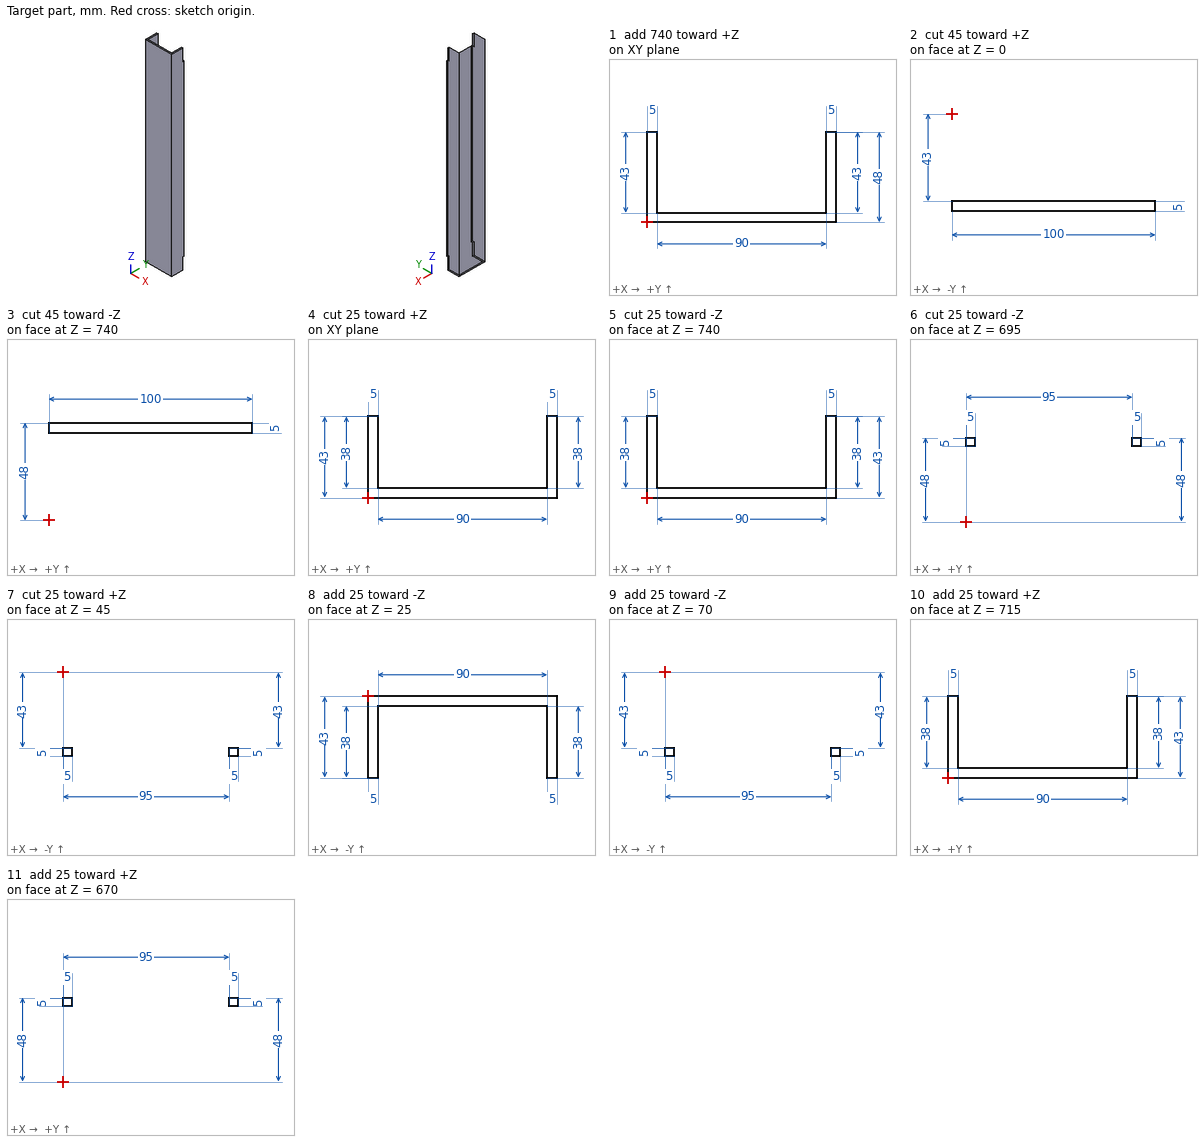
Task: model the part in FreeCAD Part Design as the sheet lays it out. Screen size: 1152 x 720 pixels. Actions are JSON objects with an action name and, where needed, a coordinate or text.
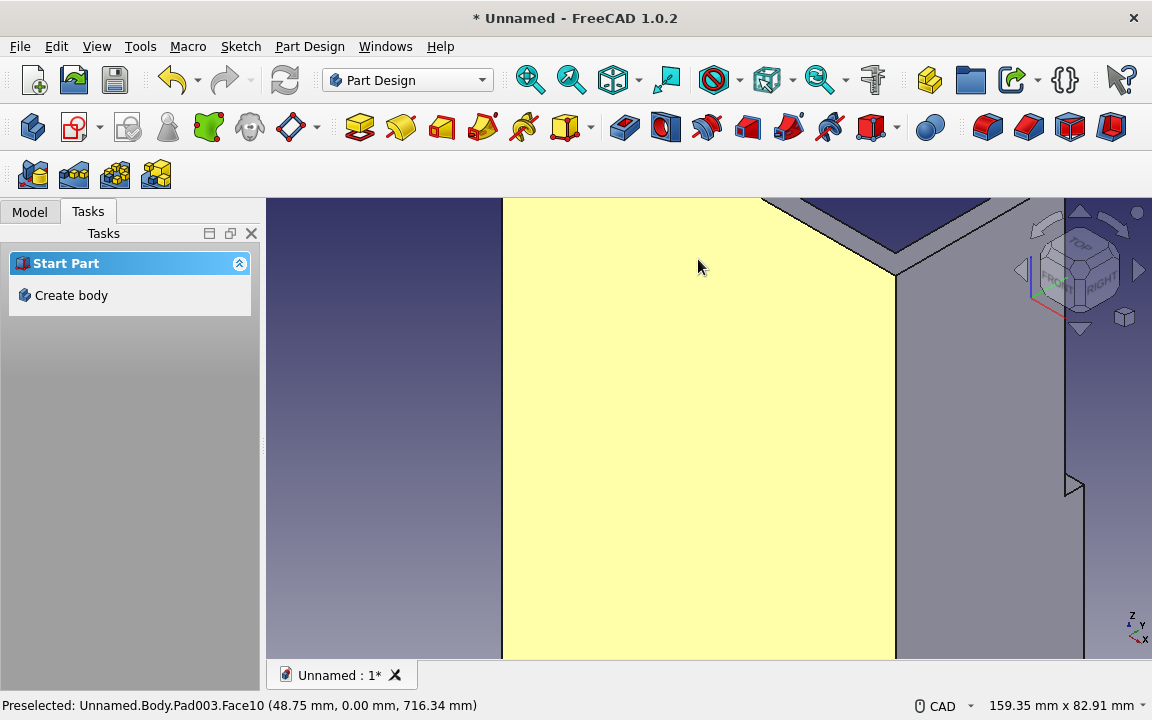
{"action": "left_click", "coordinate": [531, 80]}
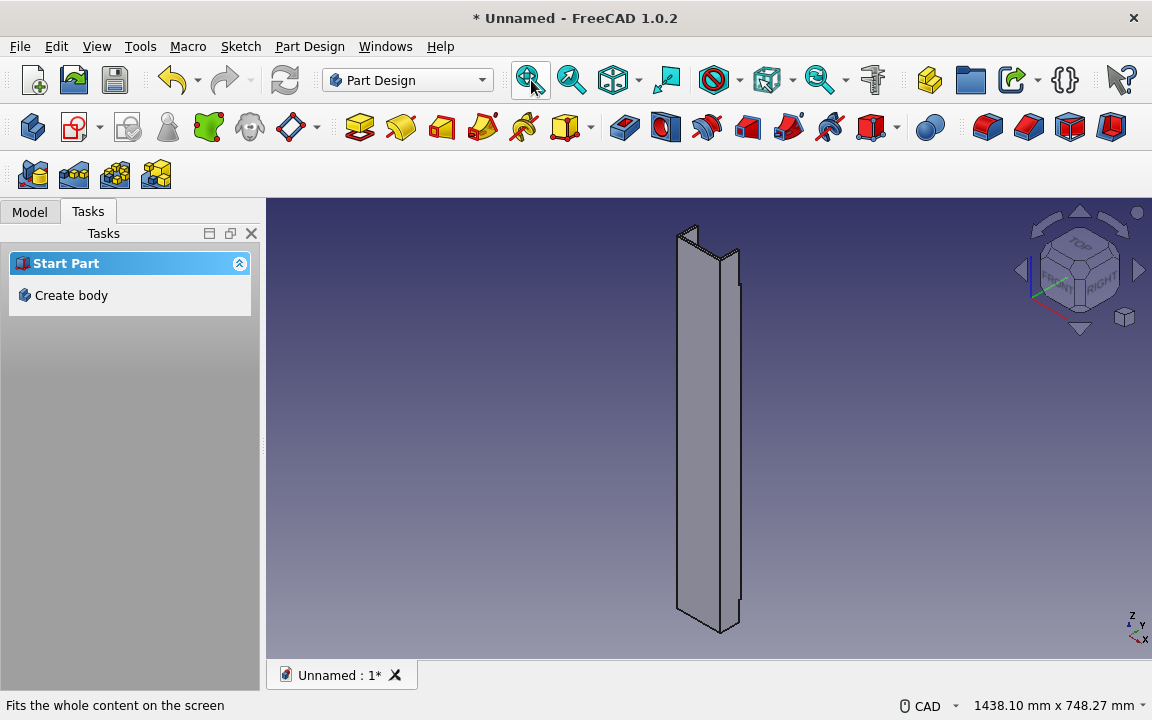
{"action": "key", "text": "2"}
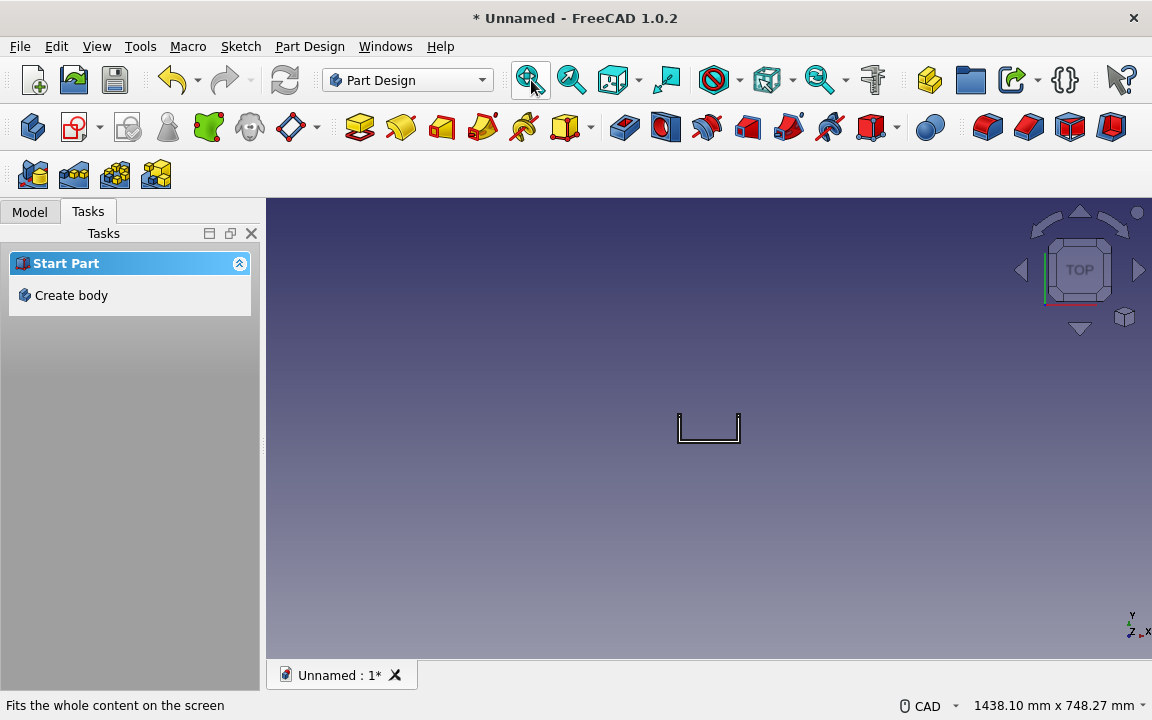
{"action": "left_click", "coordinate": [531, 80]}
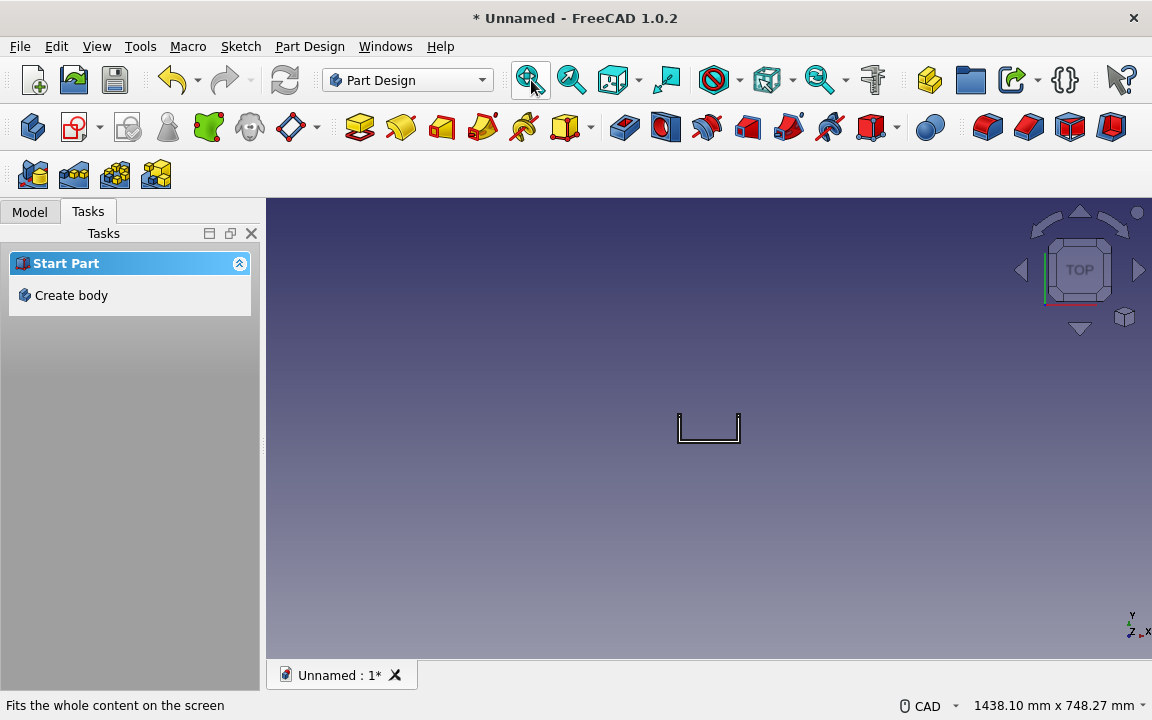
{"action": "scroll", "coordinate": [680, 414], "scroll_direction": "up", "scroll_amount": 11}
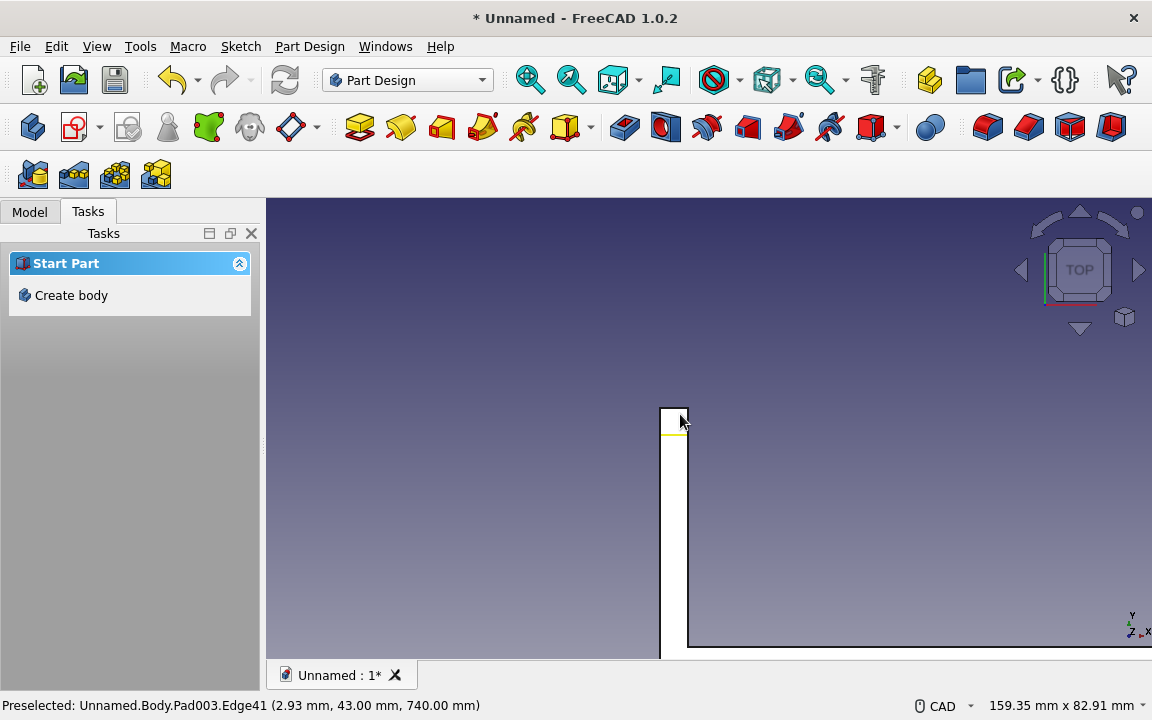
{"action": "left_click", "coordinate": [674, 421]}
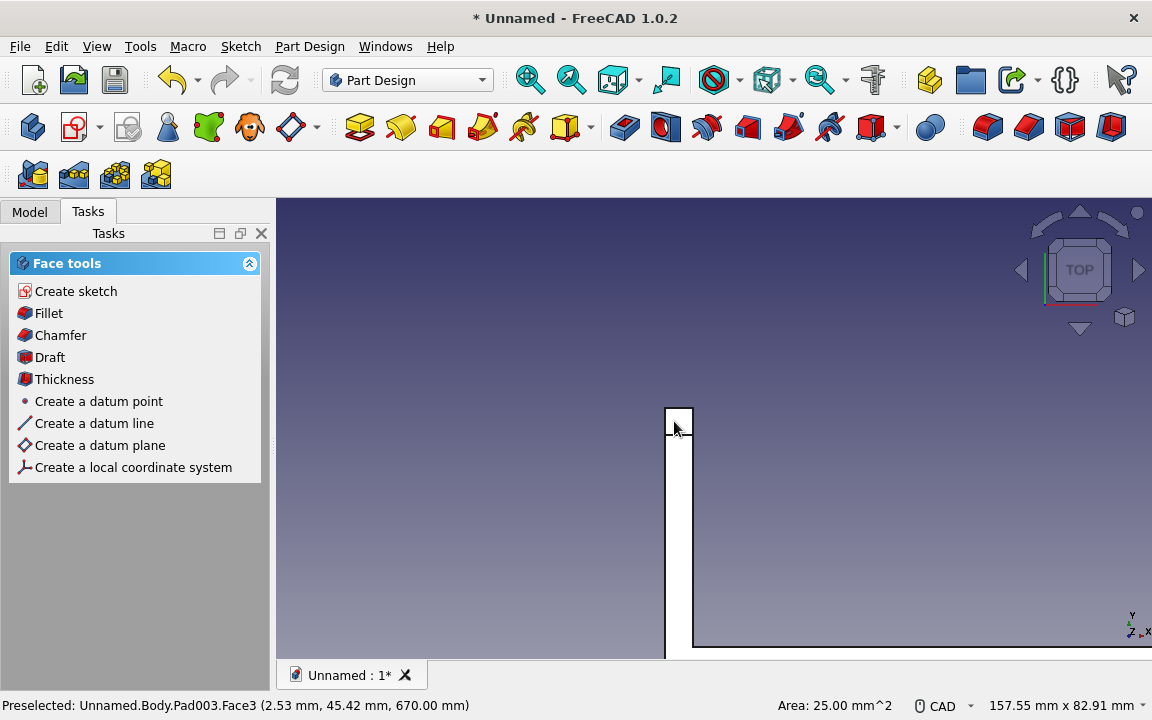
{"action": "left_click", "coordinate": [74, 128]}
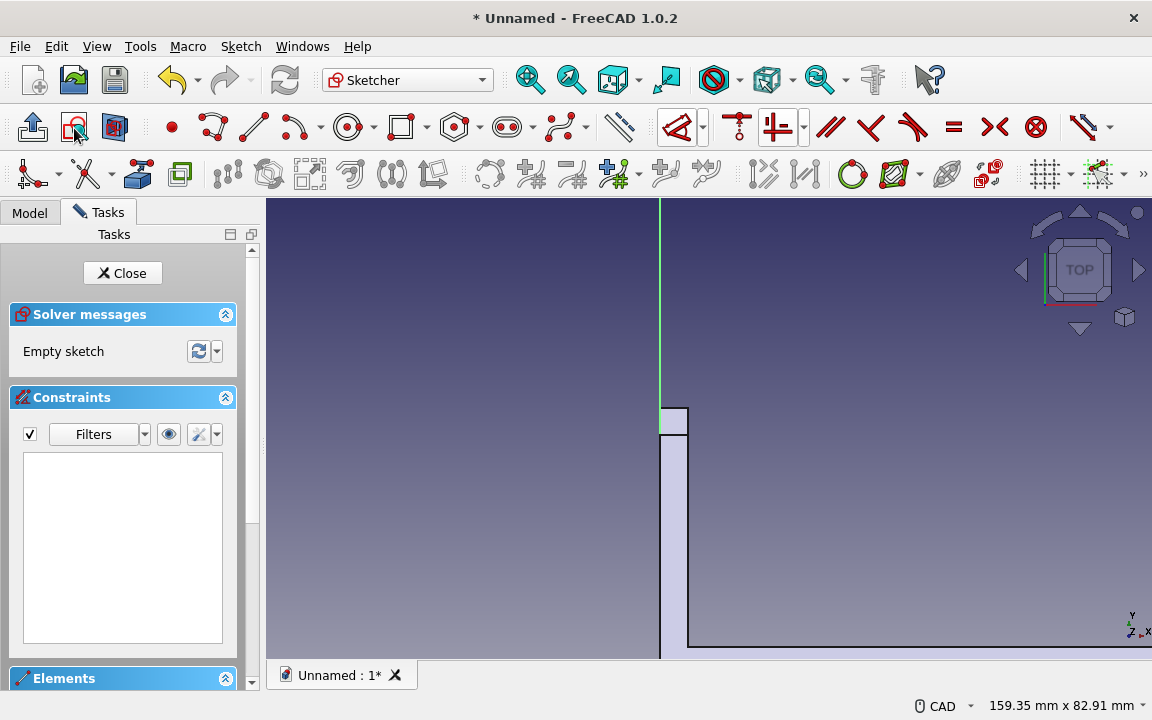
{"action": "scroll", "coordinate": [294, 226], "scroll_direction": "down", "scroll_amount": 2}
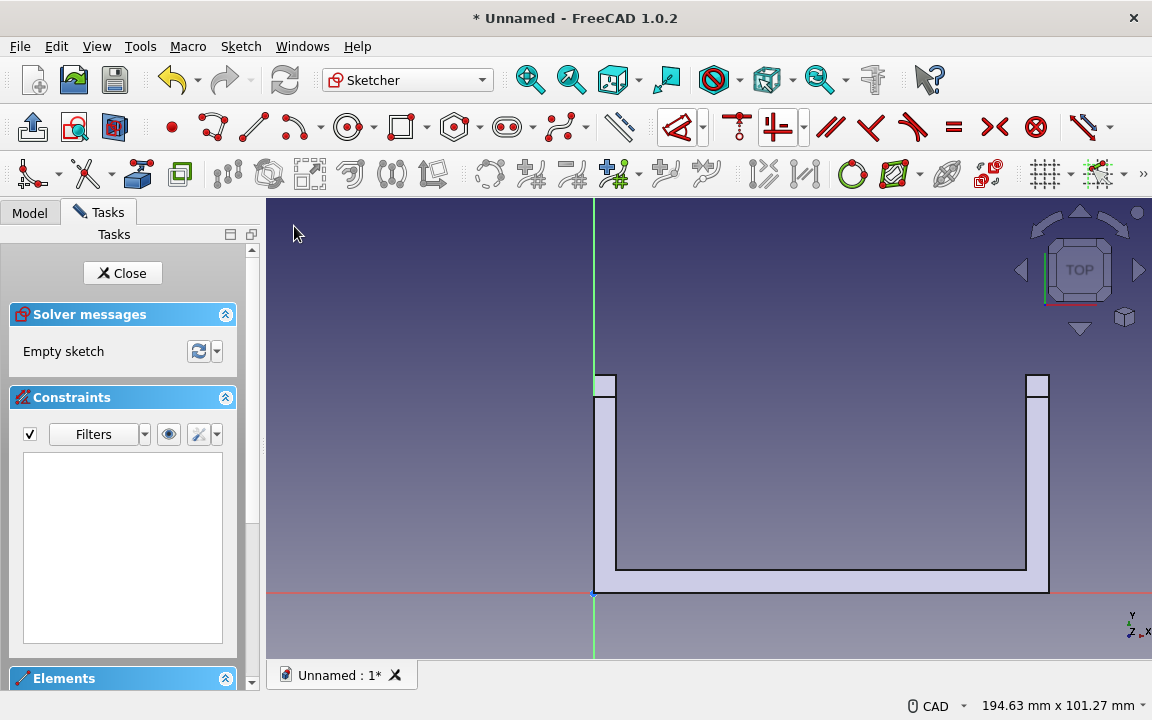
{"action": "left_click", "coordinate": [400, 128]}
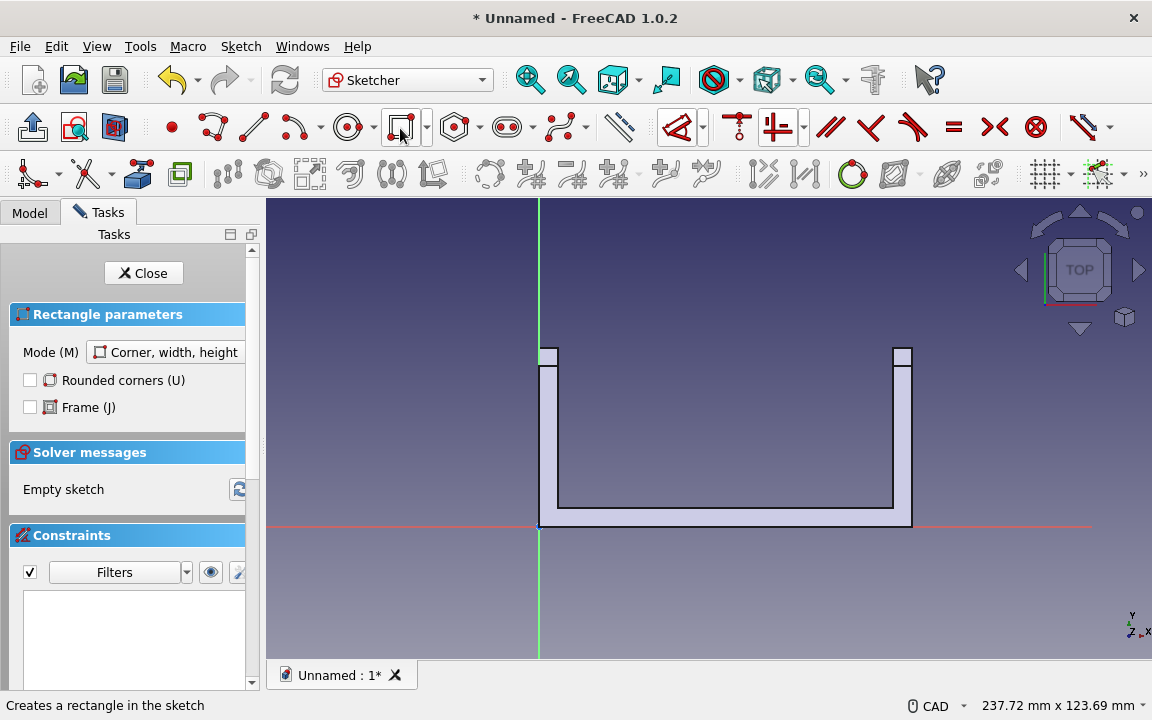
{"action": "left_click", "coordinate": [539, 348]}
{"action": "mouse_move", "coordinate": [558, 366]}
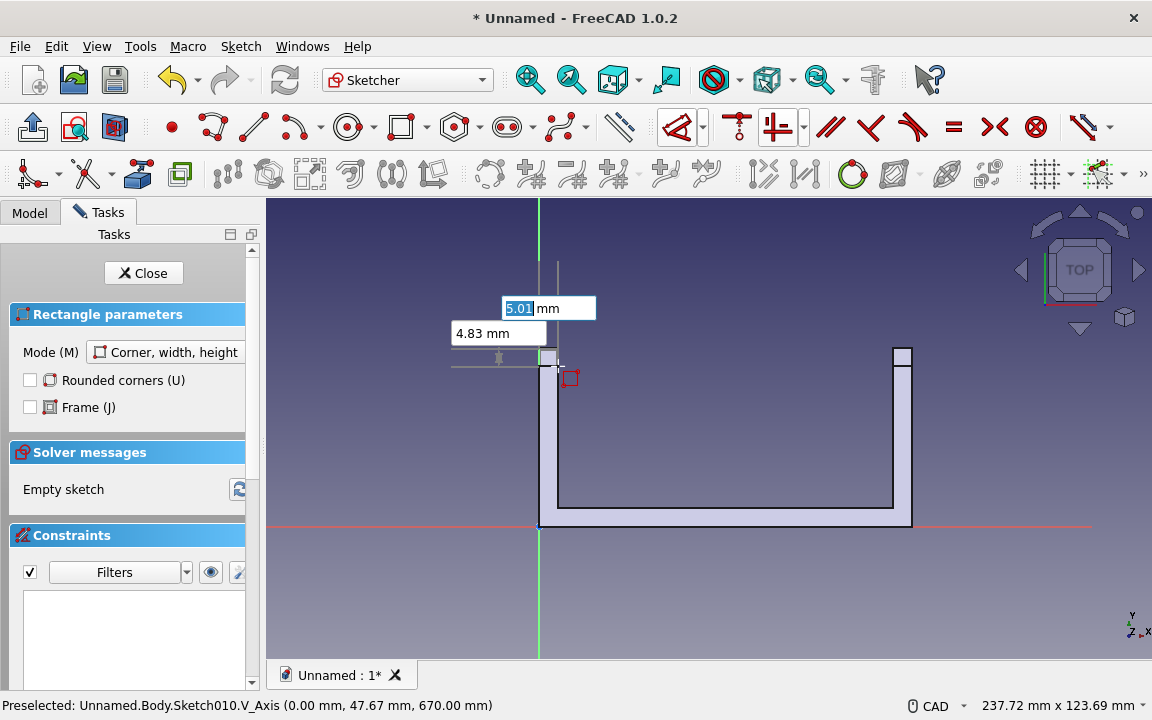
{"action": "type", "text": "5"}
{"action": "key", "text": "Tab"}
{"action": "type", "text": "5"}
{"action": "key", "text": "Return"}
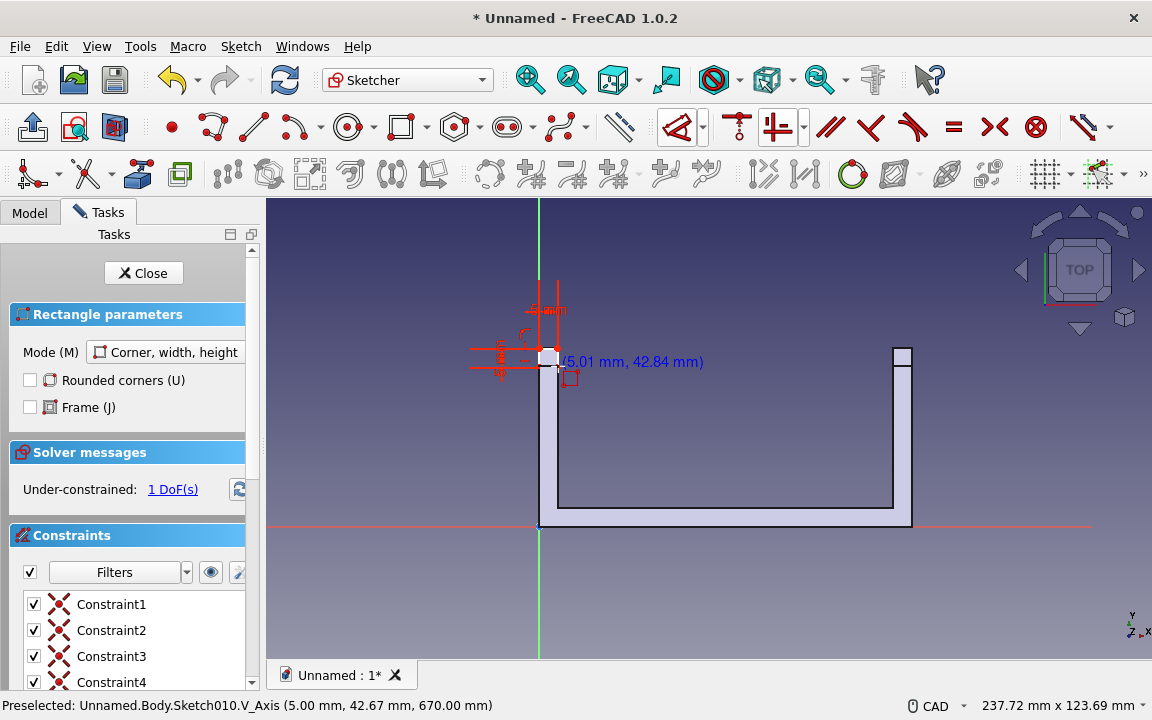
{"action": "left_click", "coordinate": [893, 348]}
{"action": "mouse_move", "coordinate": [912, 366]}